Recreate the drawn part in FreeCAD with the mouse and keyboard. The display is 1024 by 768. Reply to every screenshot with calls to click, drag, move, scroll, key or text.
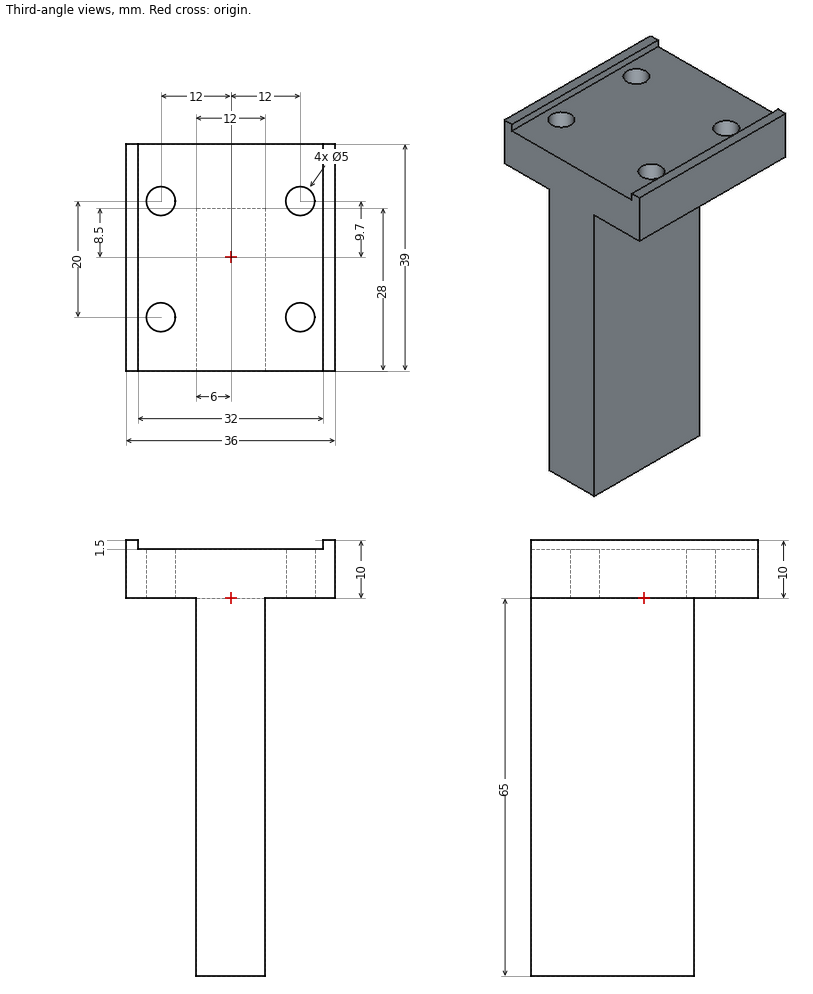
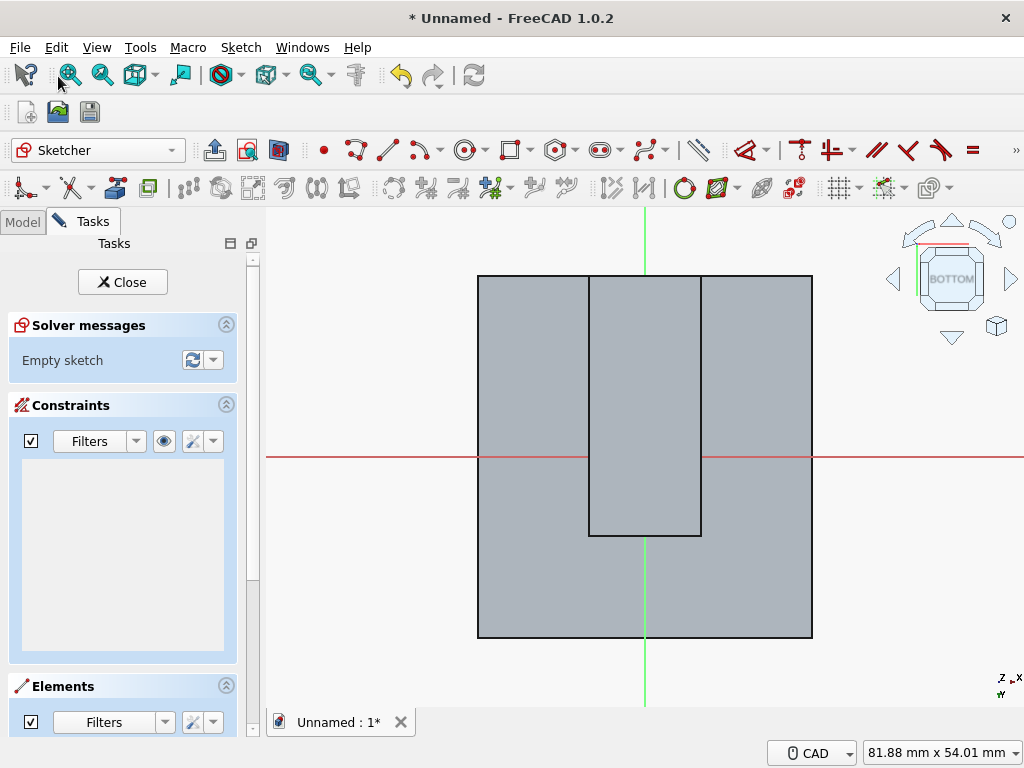
key(q)
key(s)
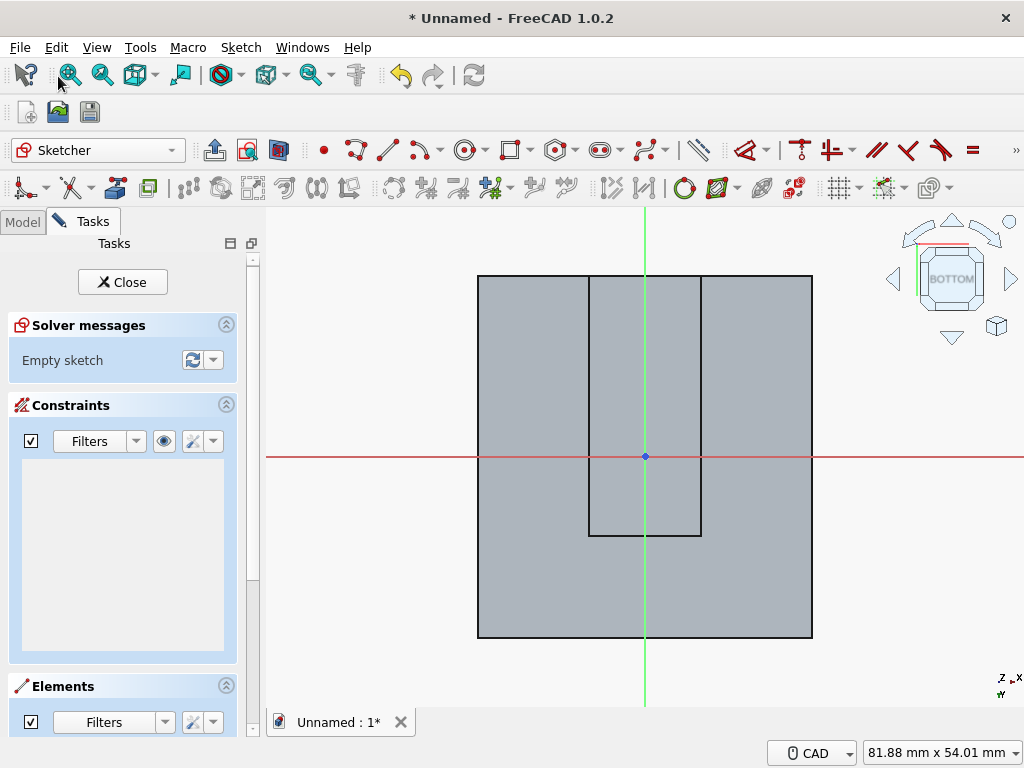
scroll(784, 449, up, 2)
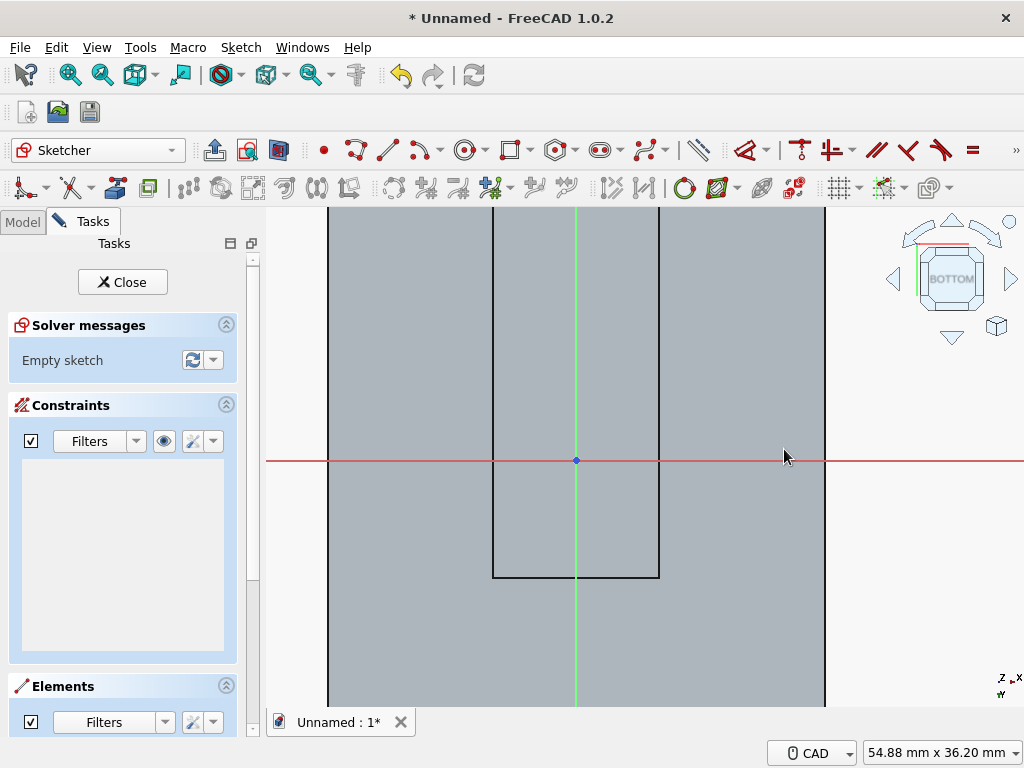
click(466, 150)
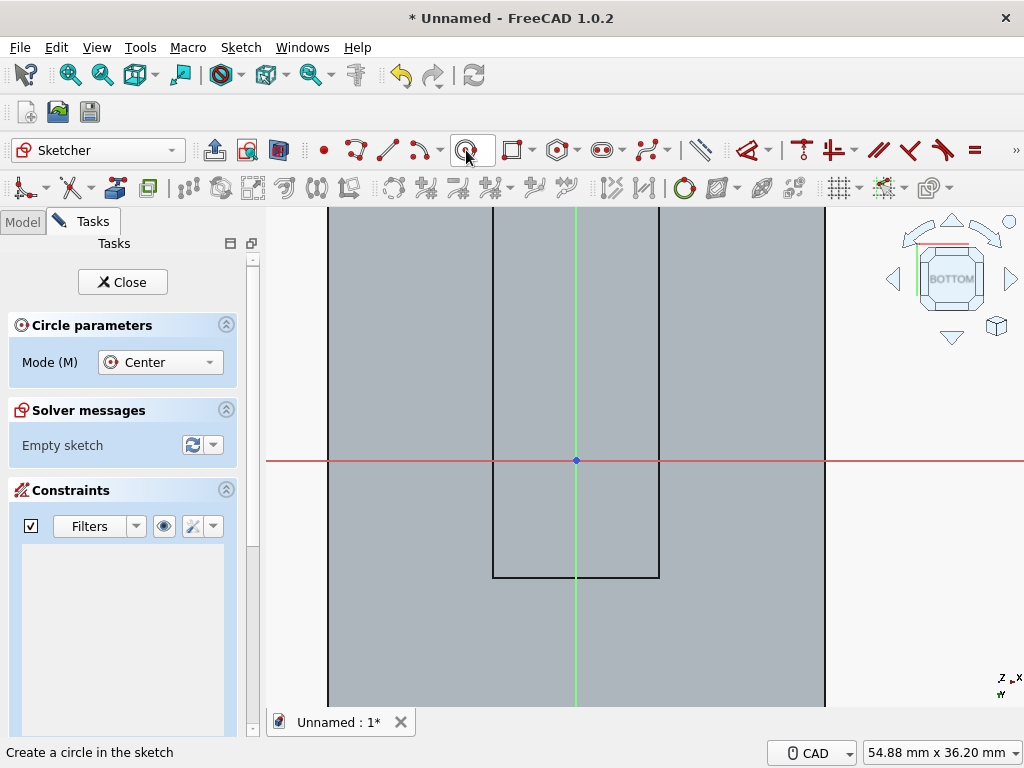
click(742, 595)
move(766, 570)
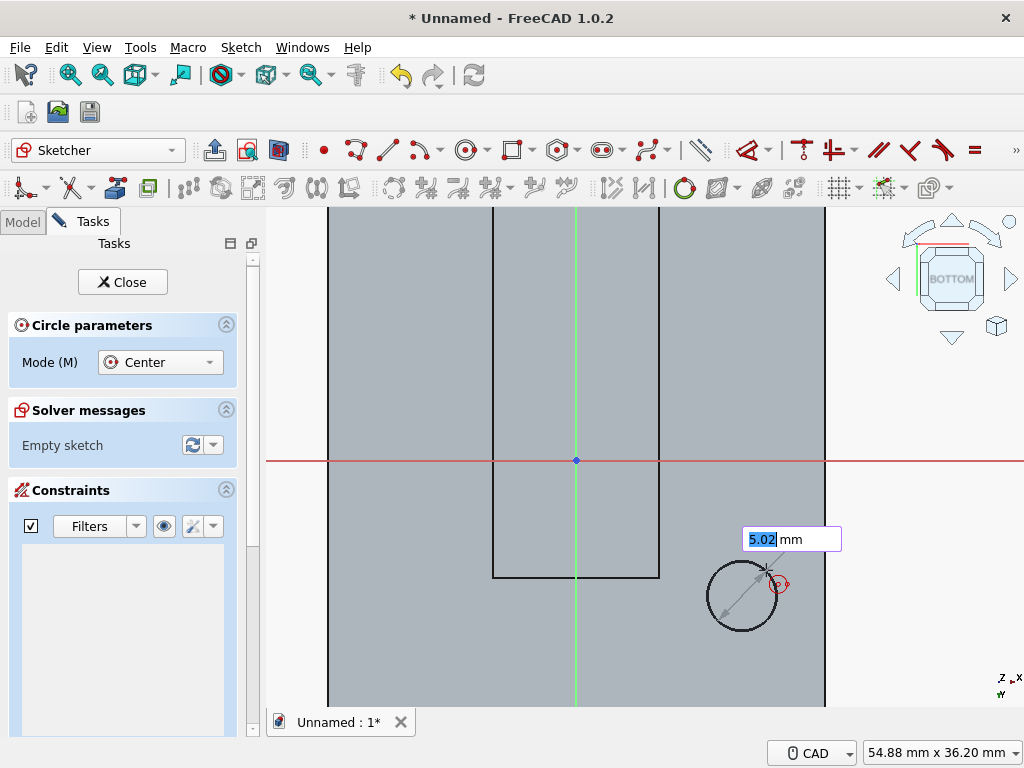
text(5)
key(Return)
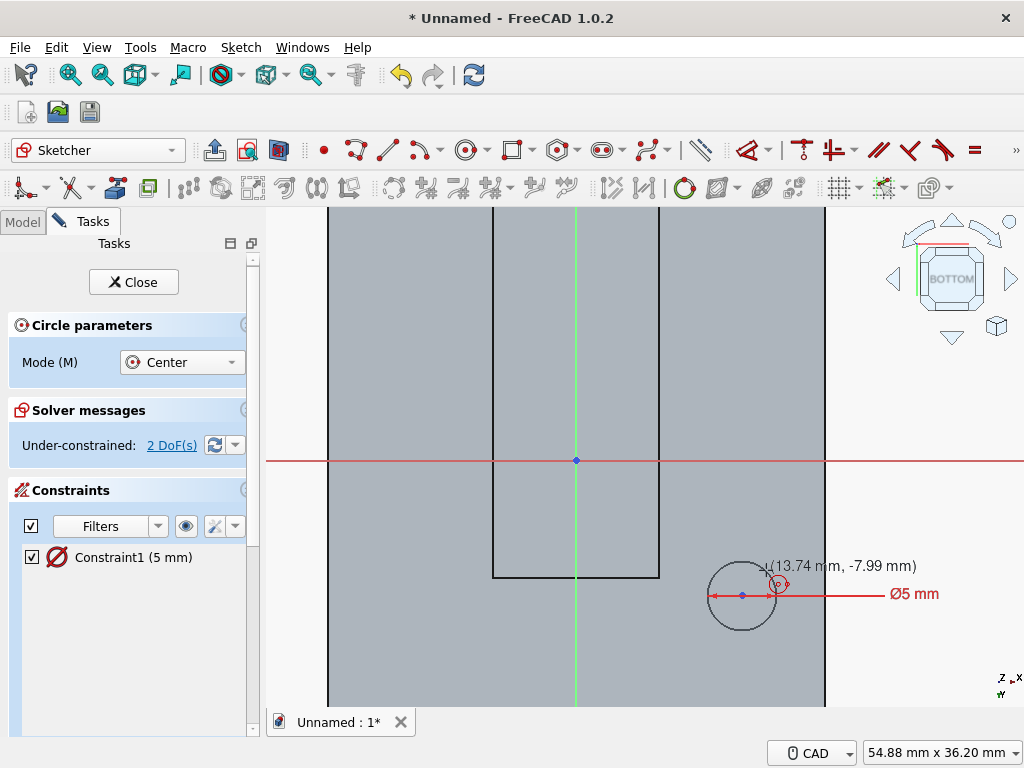
click(411, 595)
move(435, 570)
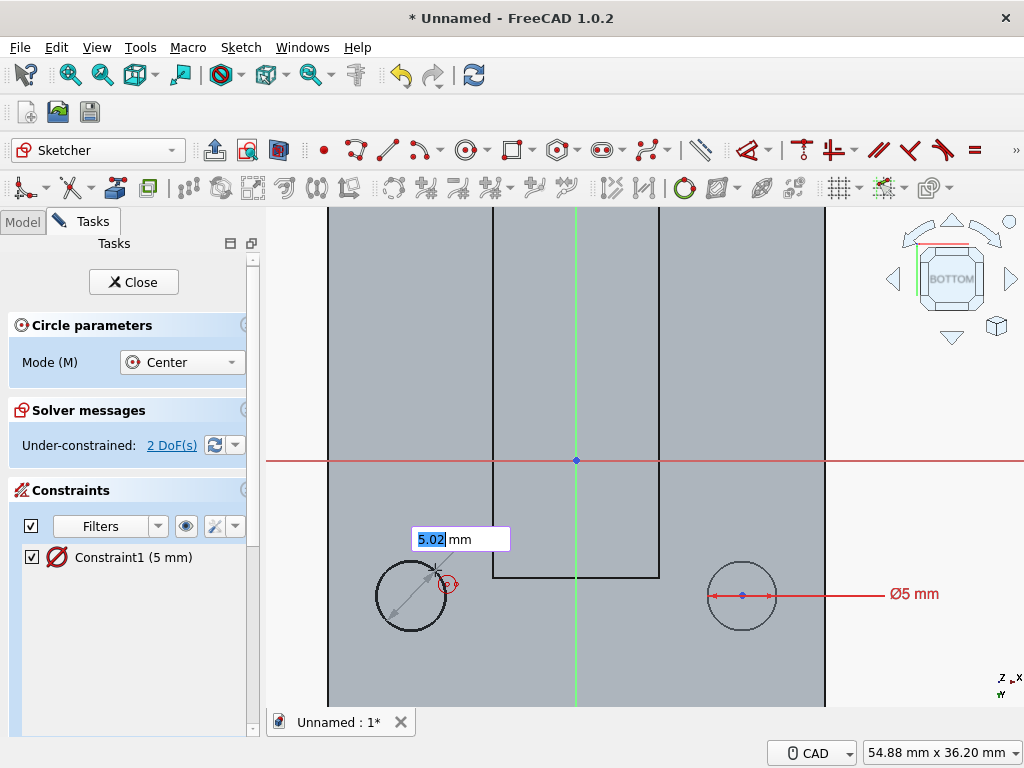
text(5)
key(Return)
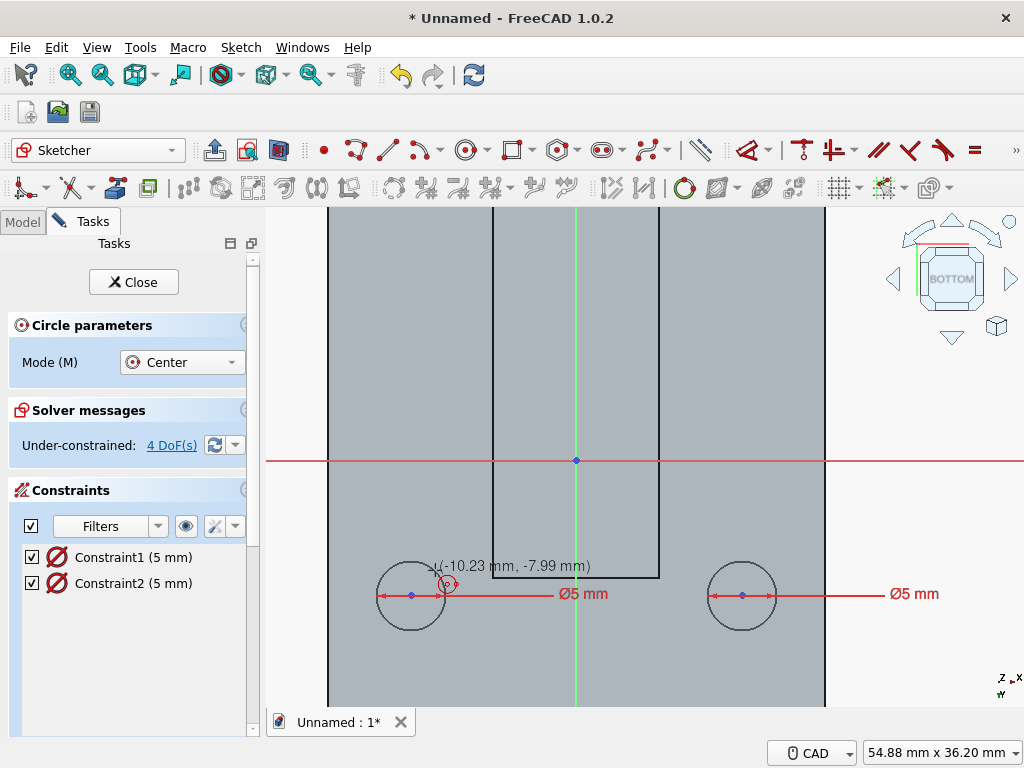
click(411, 318)
move(435, 294)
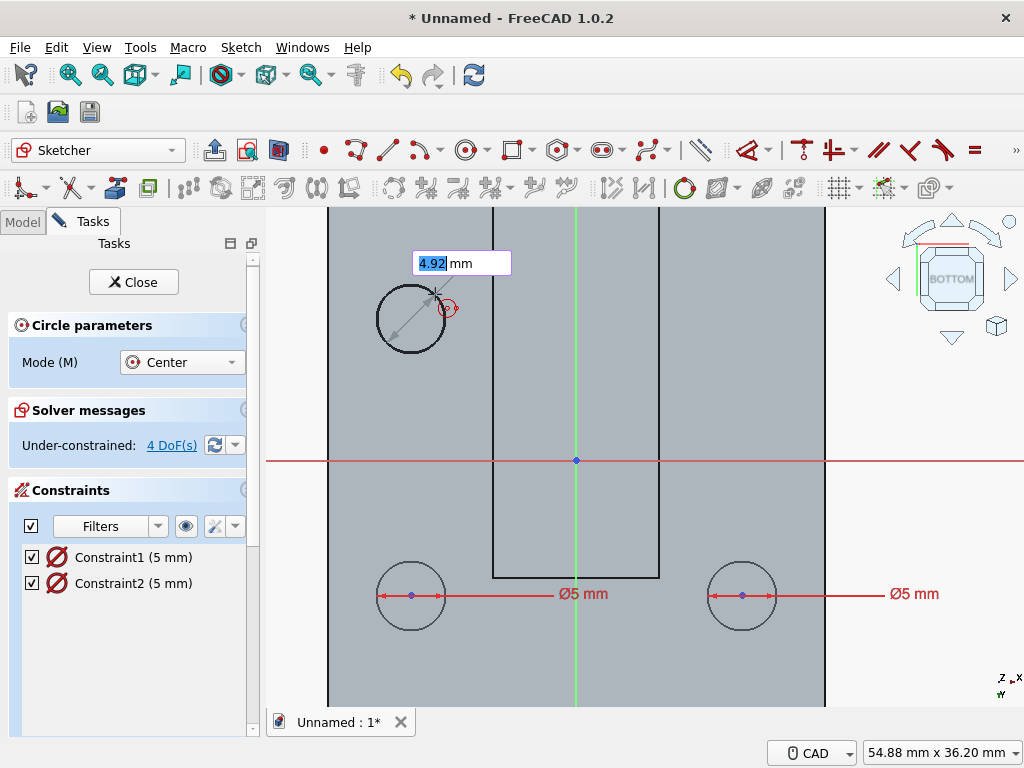
text(5)
key(Return)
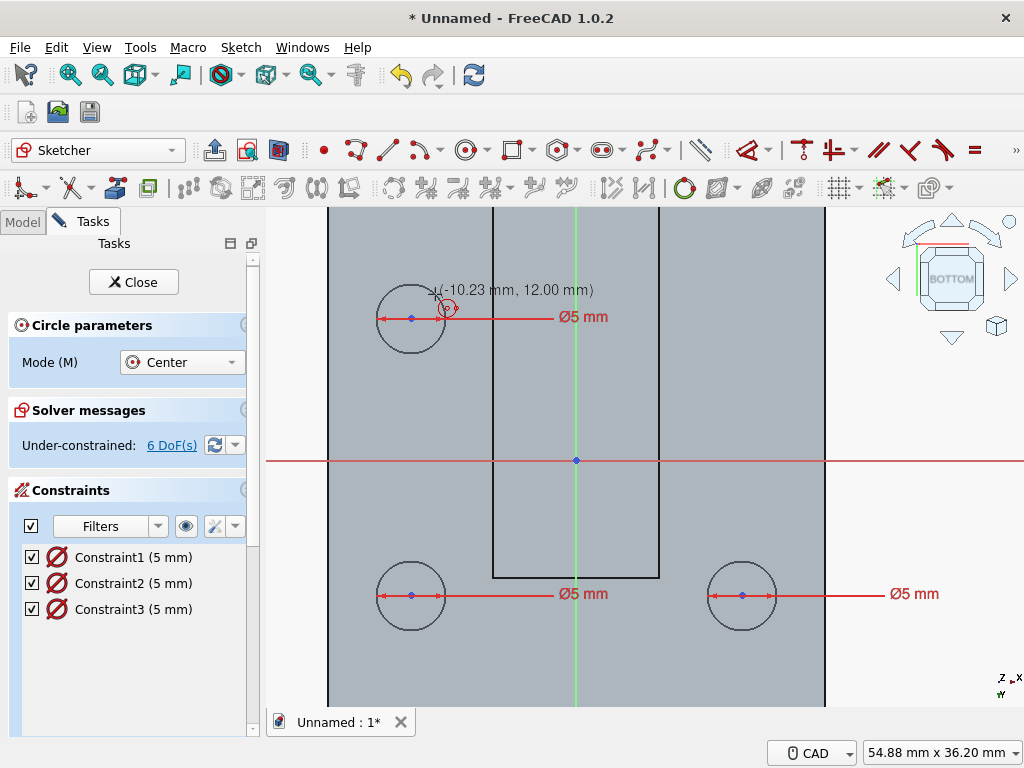
click(742, 318)
move(766, 294)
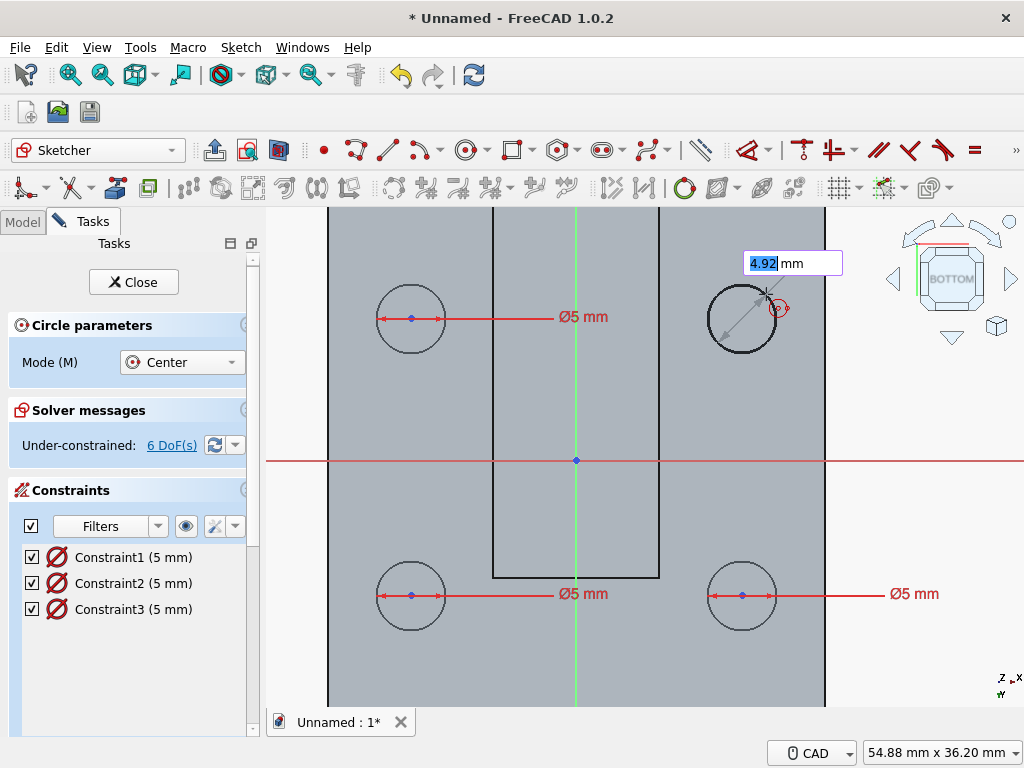
text(5)
key(Return)
key(Escape)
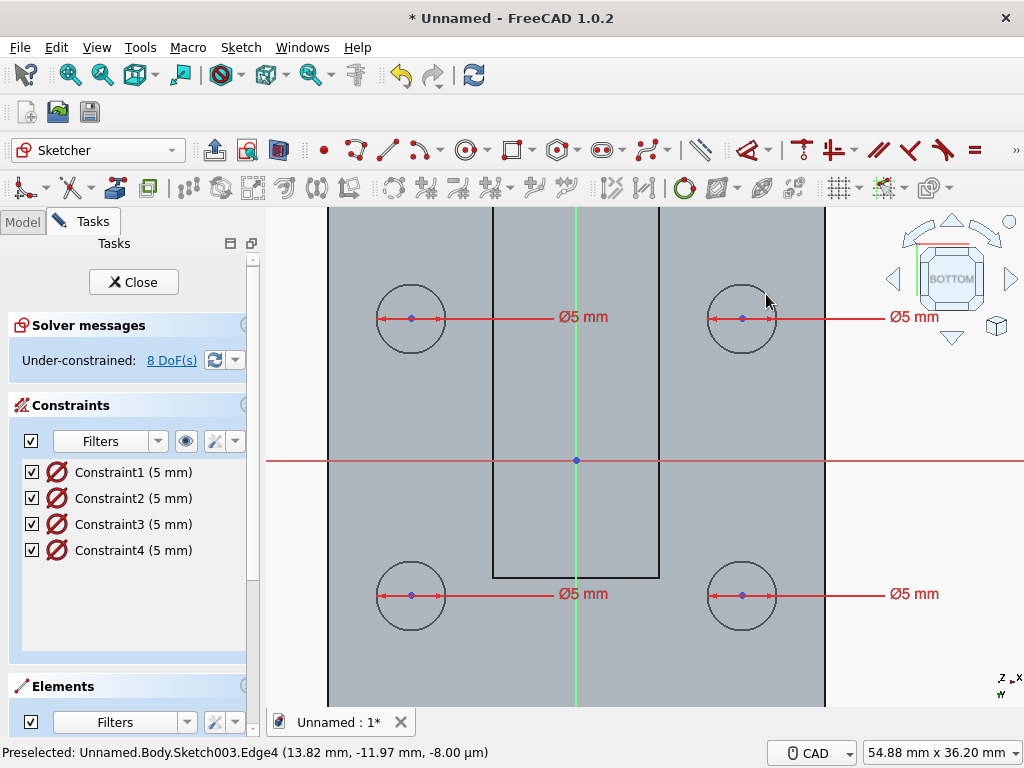
click(742, 596)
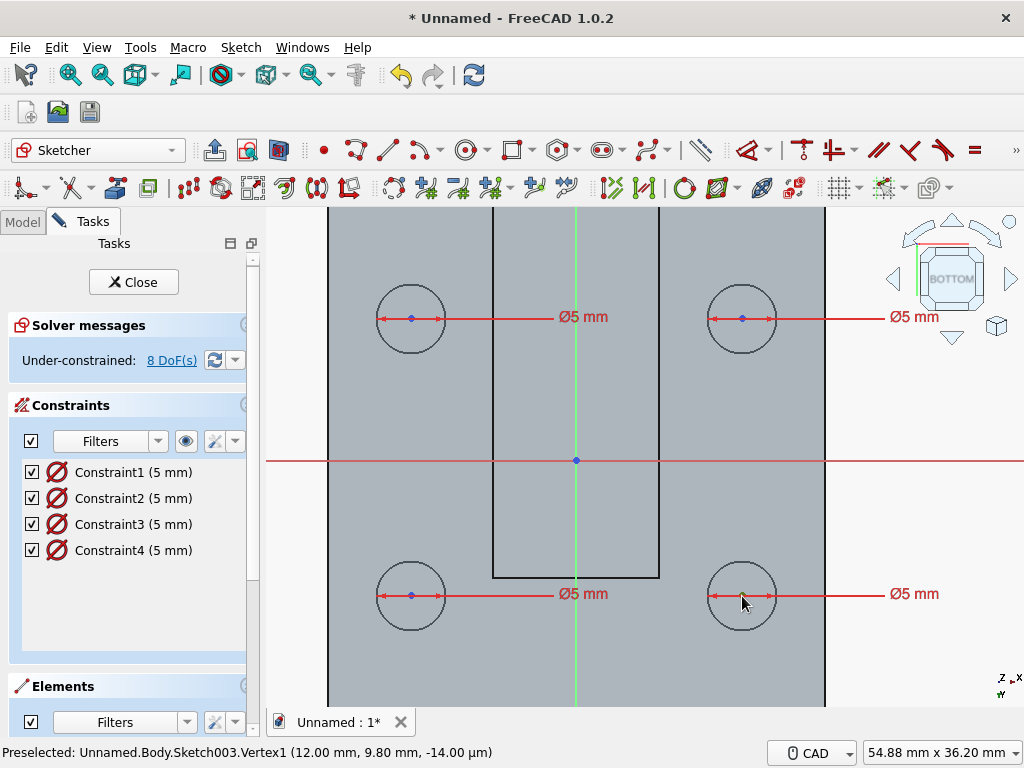
click(411, 596)